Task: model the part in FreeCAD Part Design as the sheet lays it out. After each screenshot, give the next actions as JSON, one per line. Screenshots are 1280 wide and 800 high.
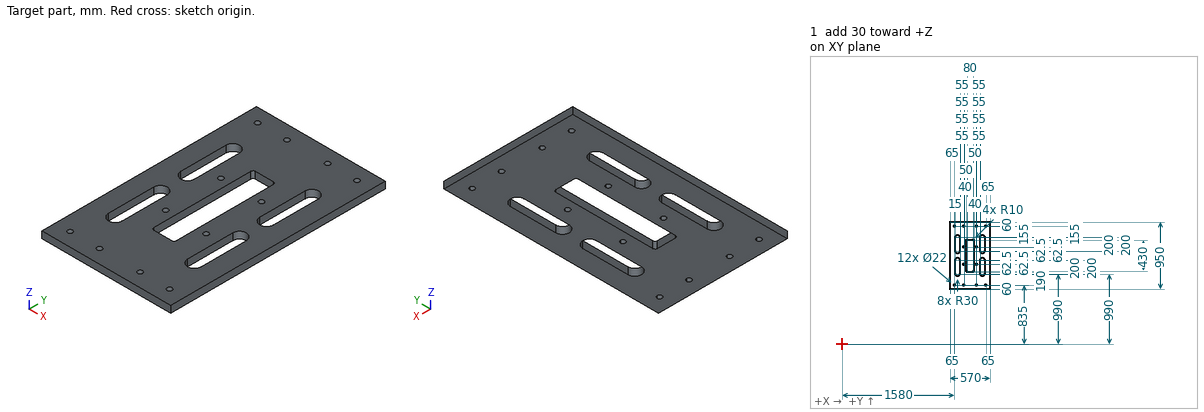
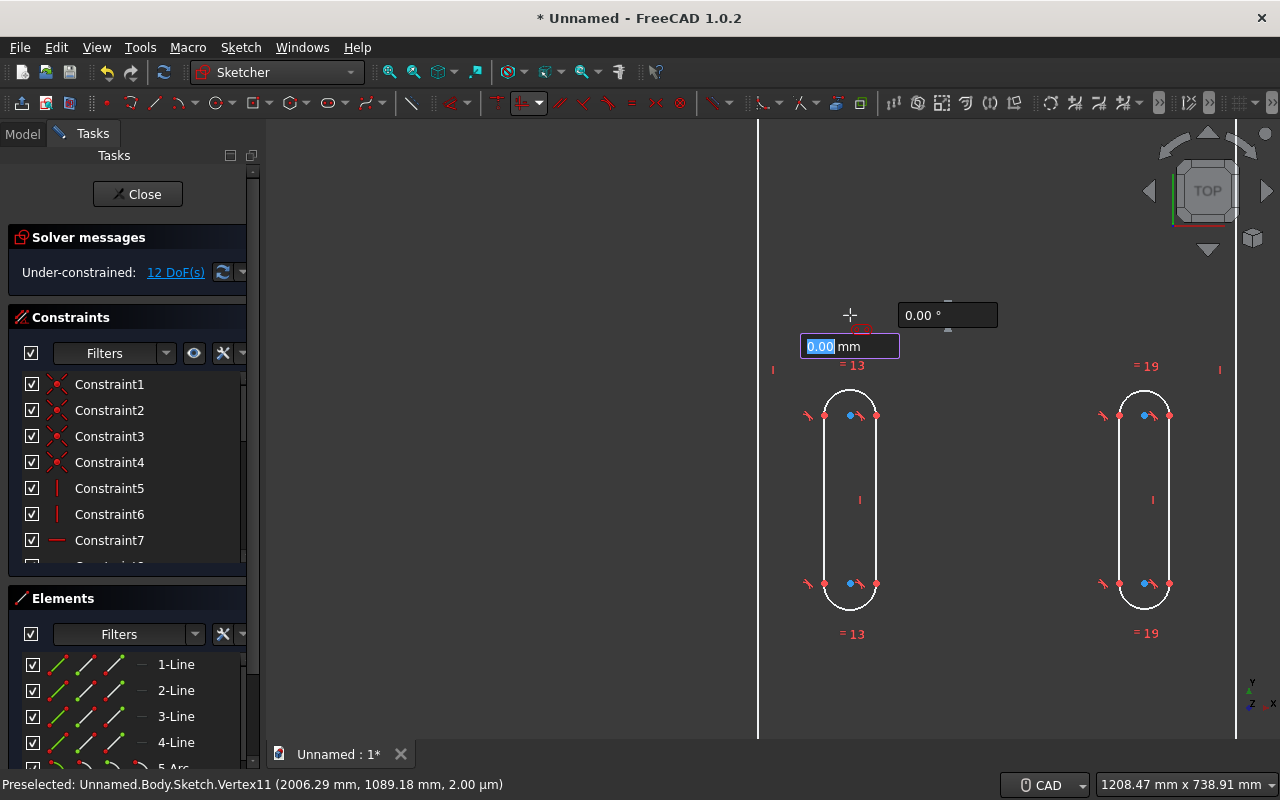
{"action": "scroll", "coordinate": [852, 316], "scroll_direction": "down", "scroll_amount": 6}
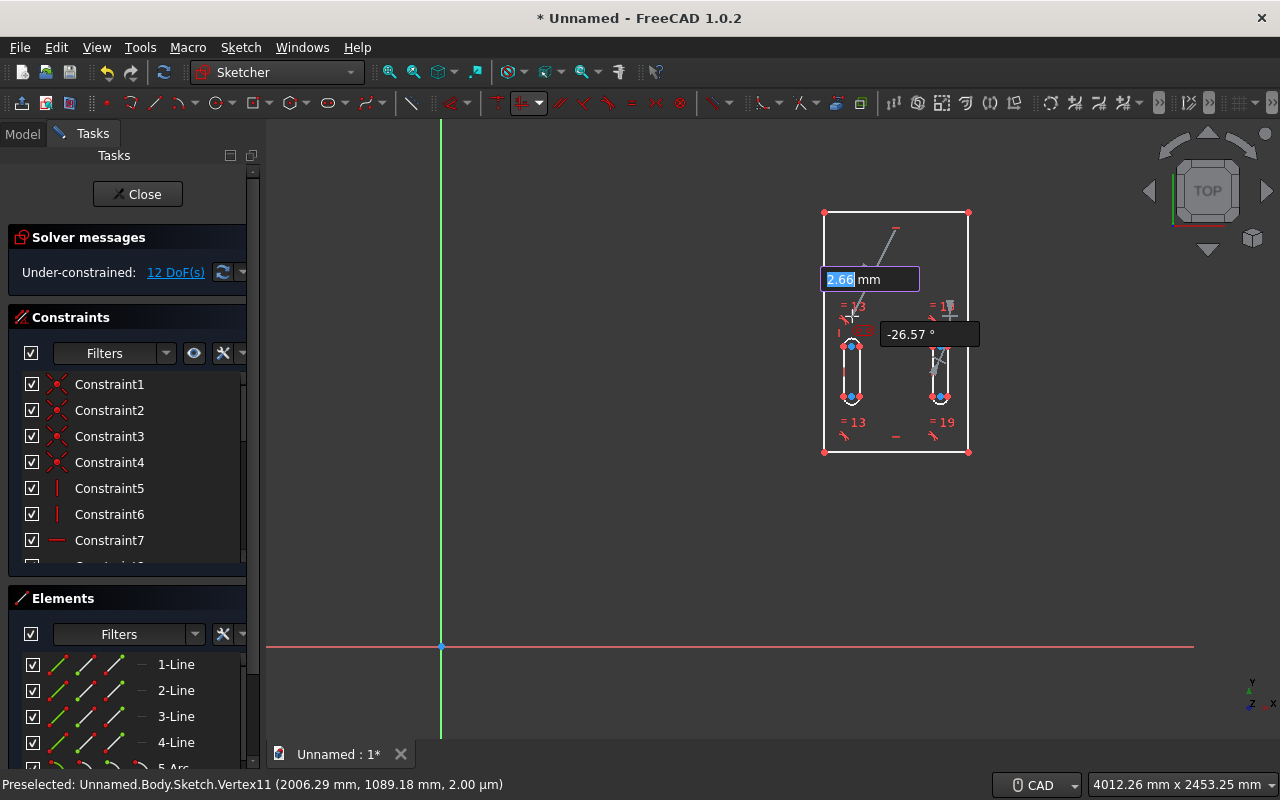
{"action": "left_click", "coordinate": [852, 265]}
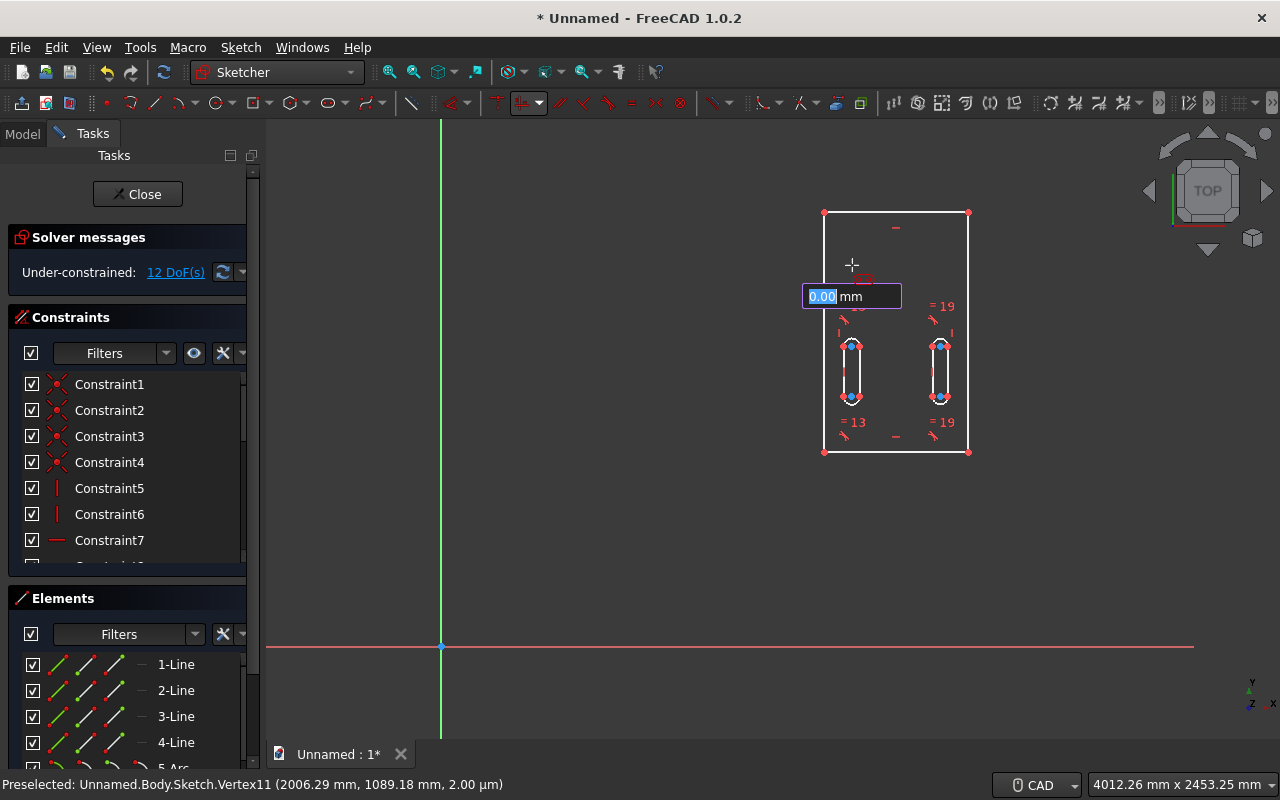
{"action": "scroll", "coordinate": [860, 291], "scroll_direction": "up", "scroll_amount": 4}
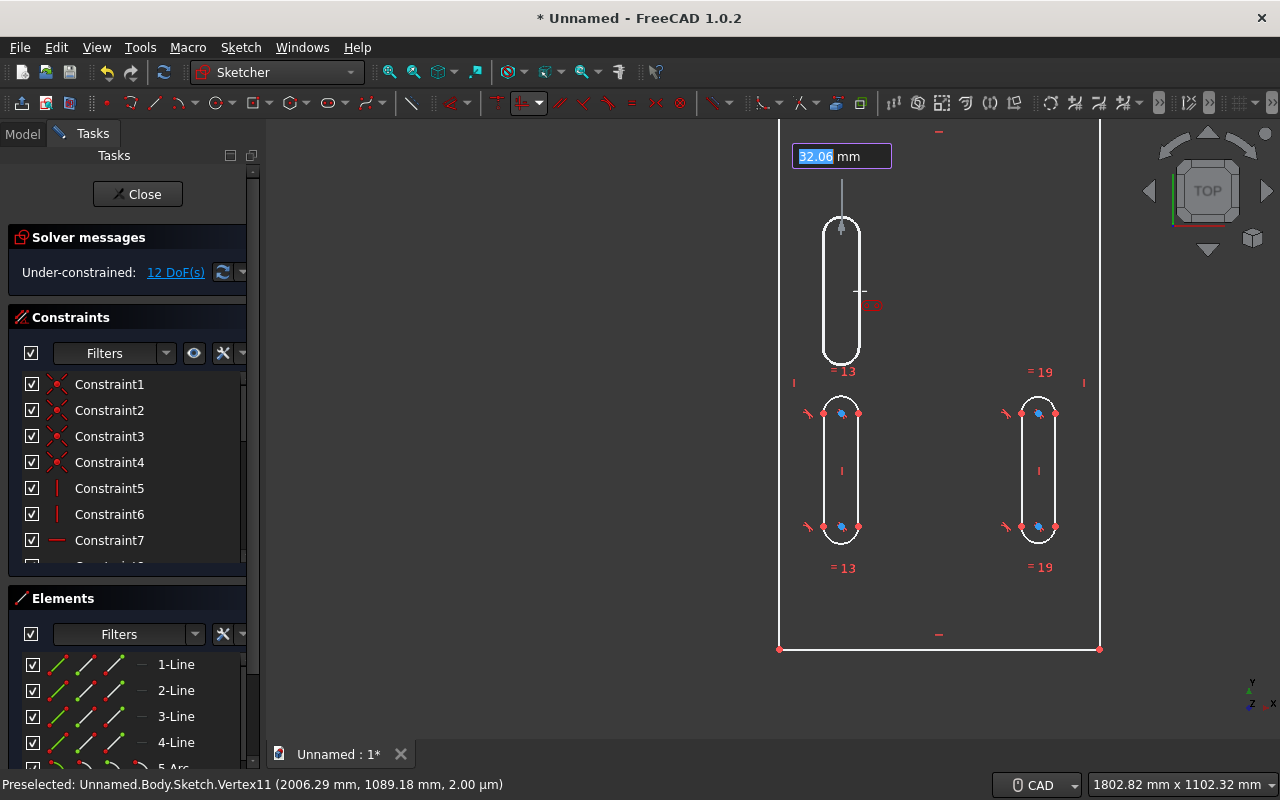
{"action": "left_click", "coordinate": [858, 290]}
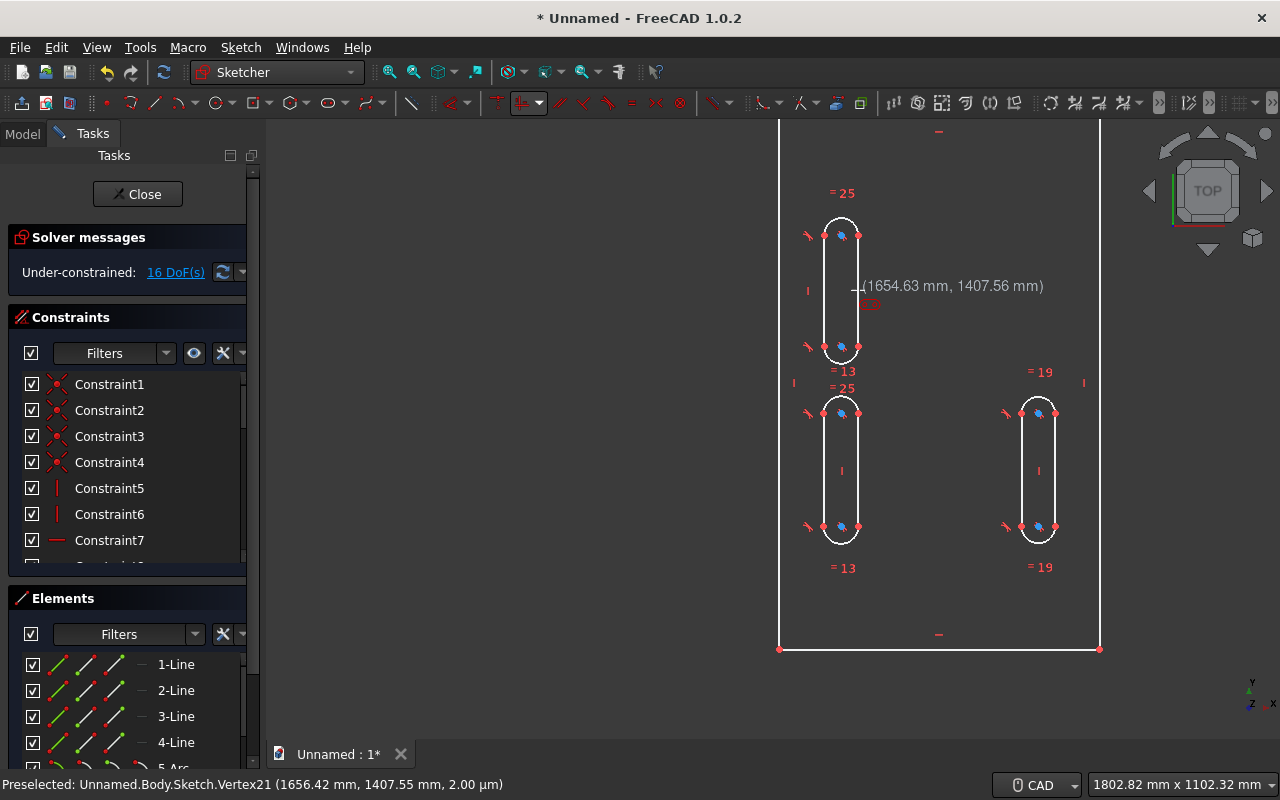
{"action": "left_click", "coordinate": [156, 104]}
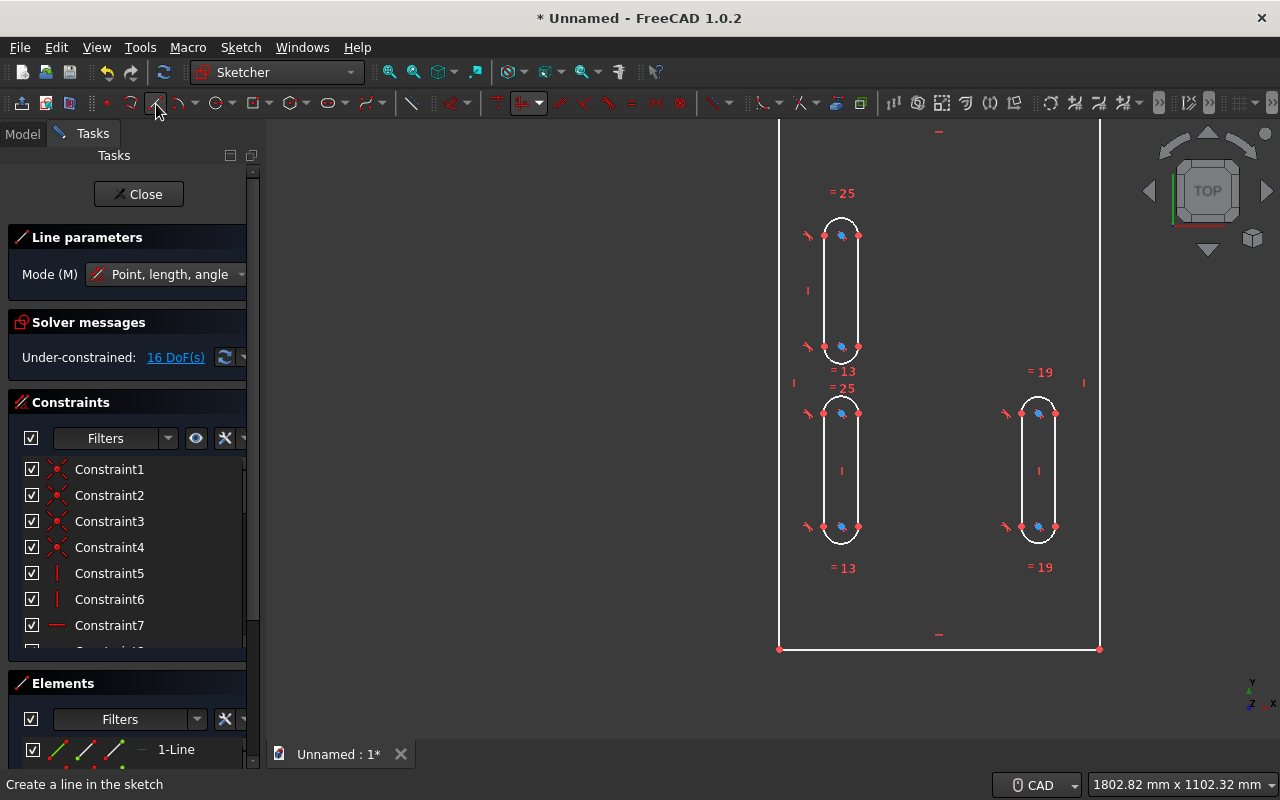
{"action": "left_click", "coordinate": [962, 506]}
{"action": "left_click", "coordinate": [917, 506]}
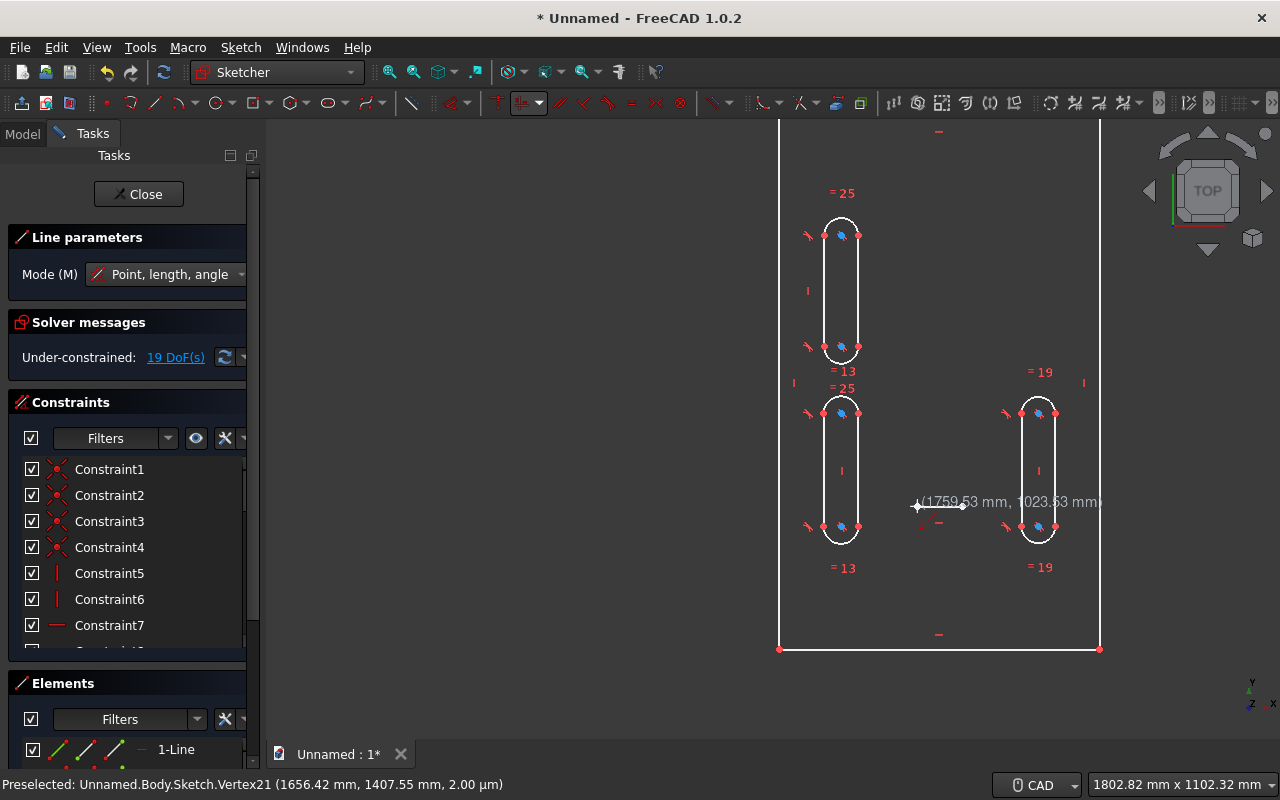
{"action": "scroll", "coordinate": [912, 501], "scroll_direction": "up", "scroll_amount": 4}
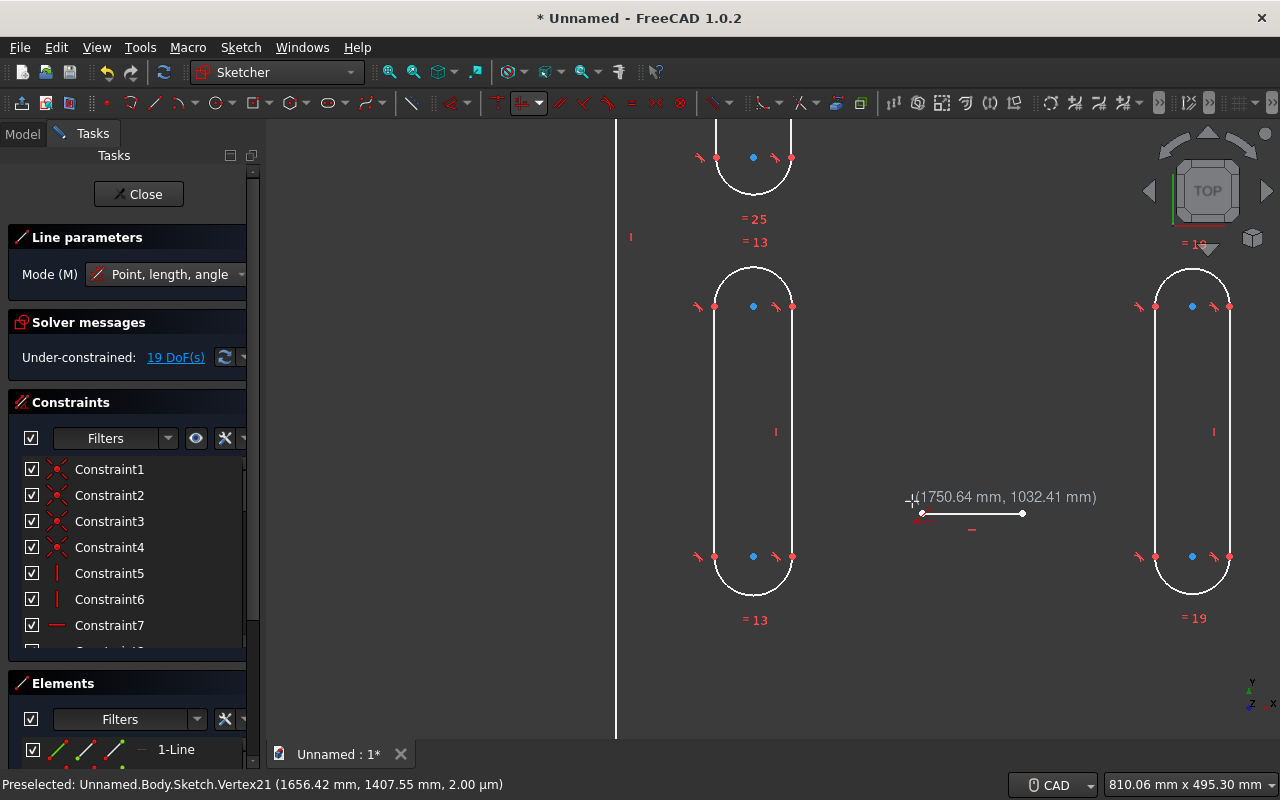
{"action": "left_click", "coordinate": [910, 499]}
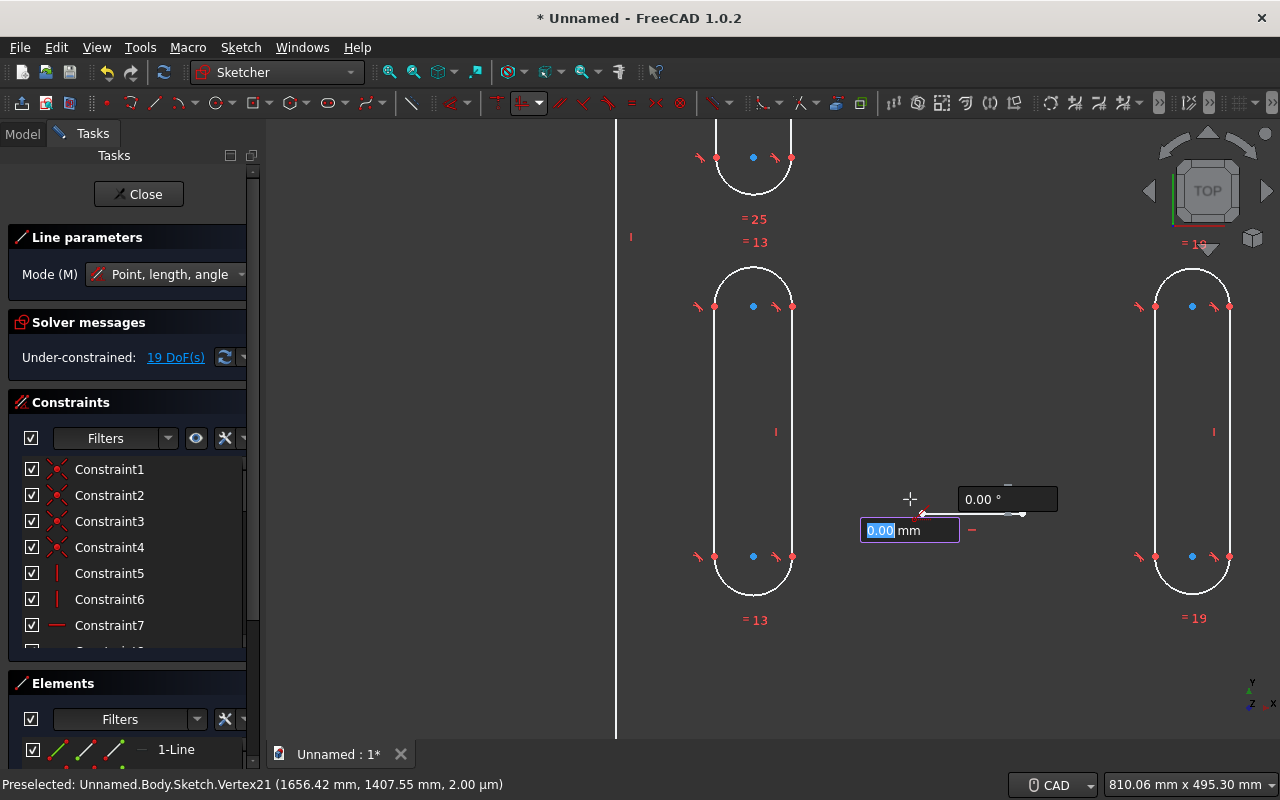
{"action": "scroll", "coordinate": [876, 357], "scroll_direction": "down", "scroll_amount": 8}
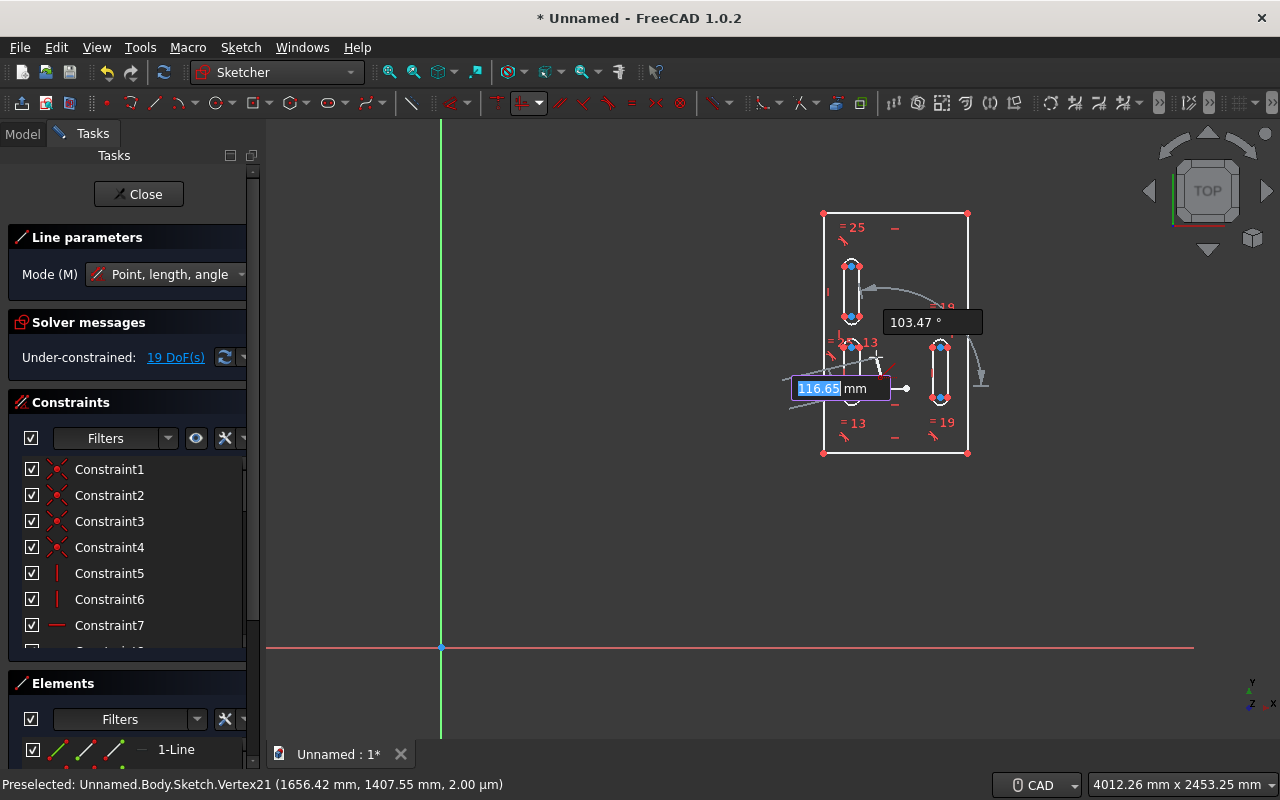
{"action": "left_click", "coordinate": [883, 277]}